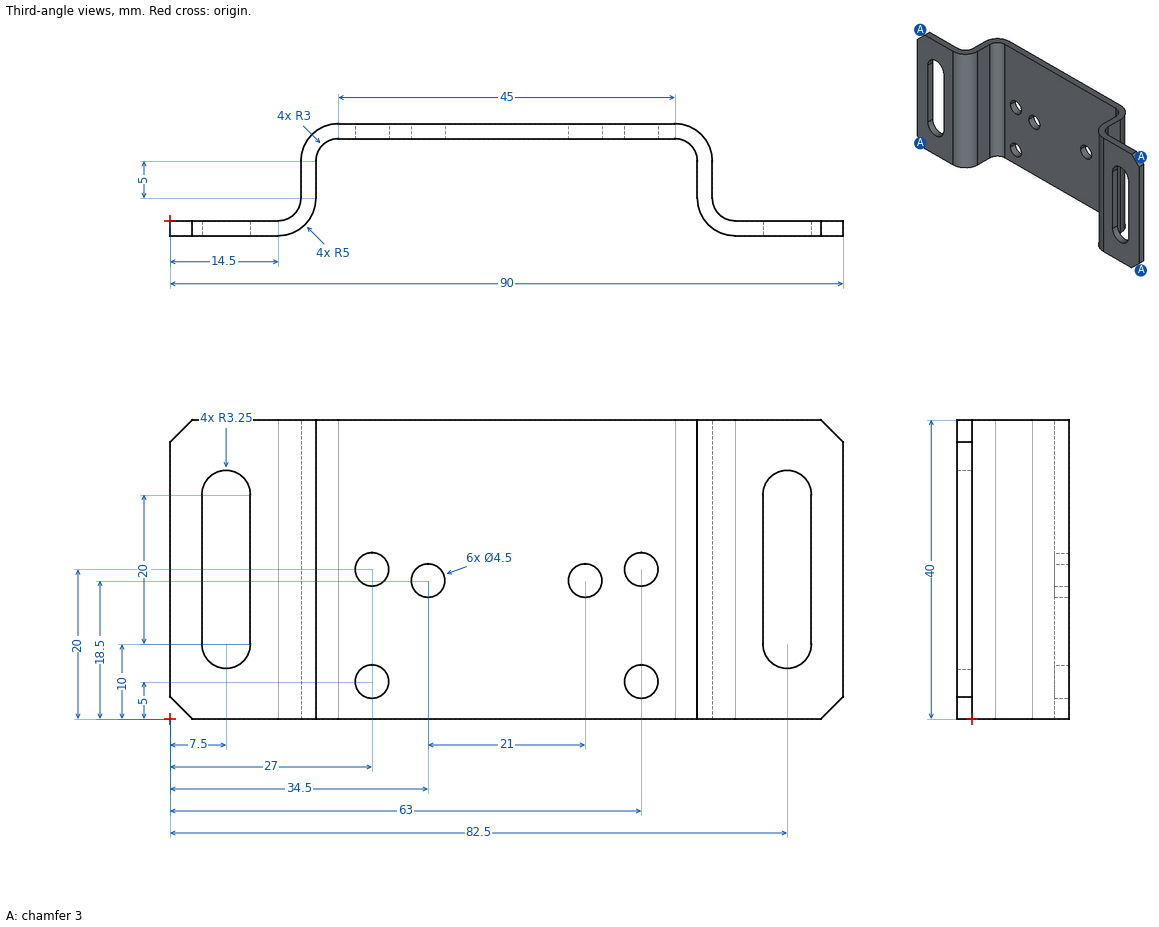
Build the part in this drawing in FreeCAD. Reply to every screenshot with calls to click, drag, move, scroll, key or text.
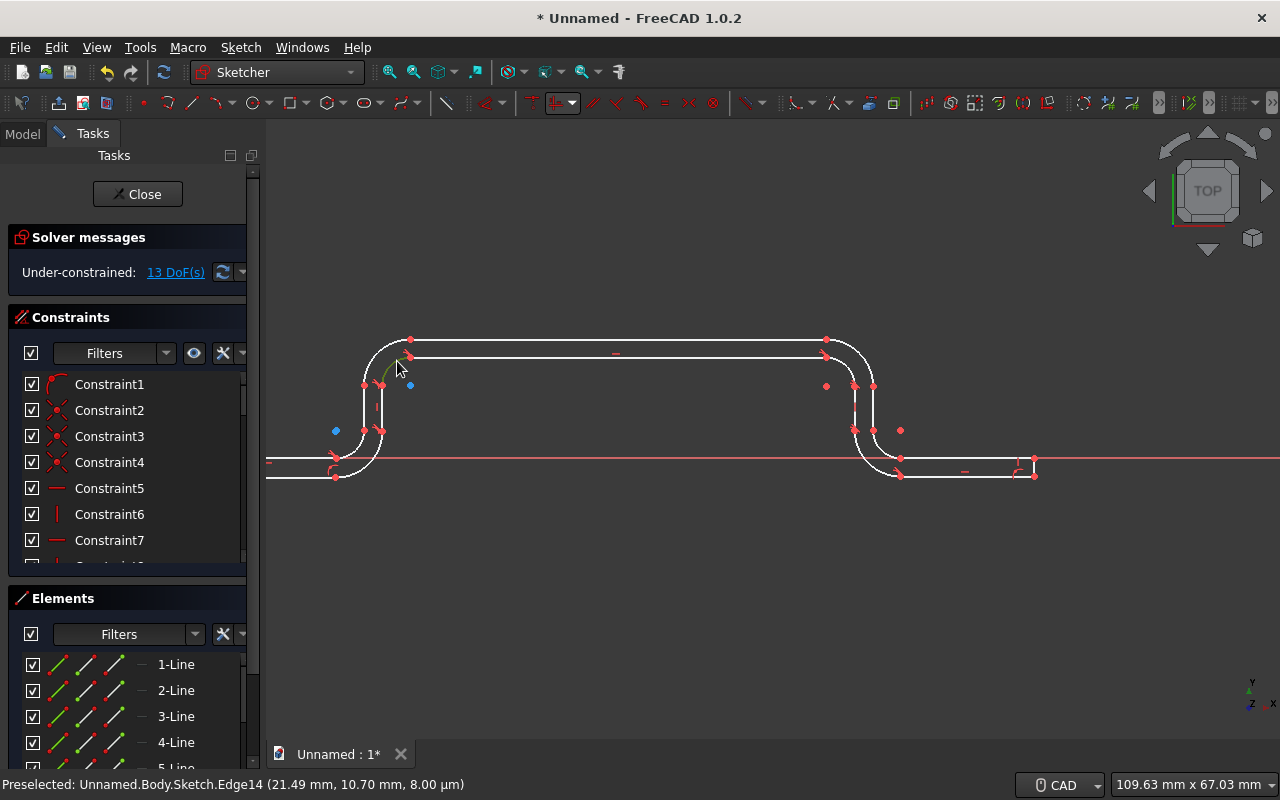
click(389, 345)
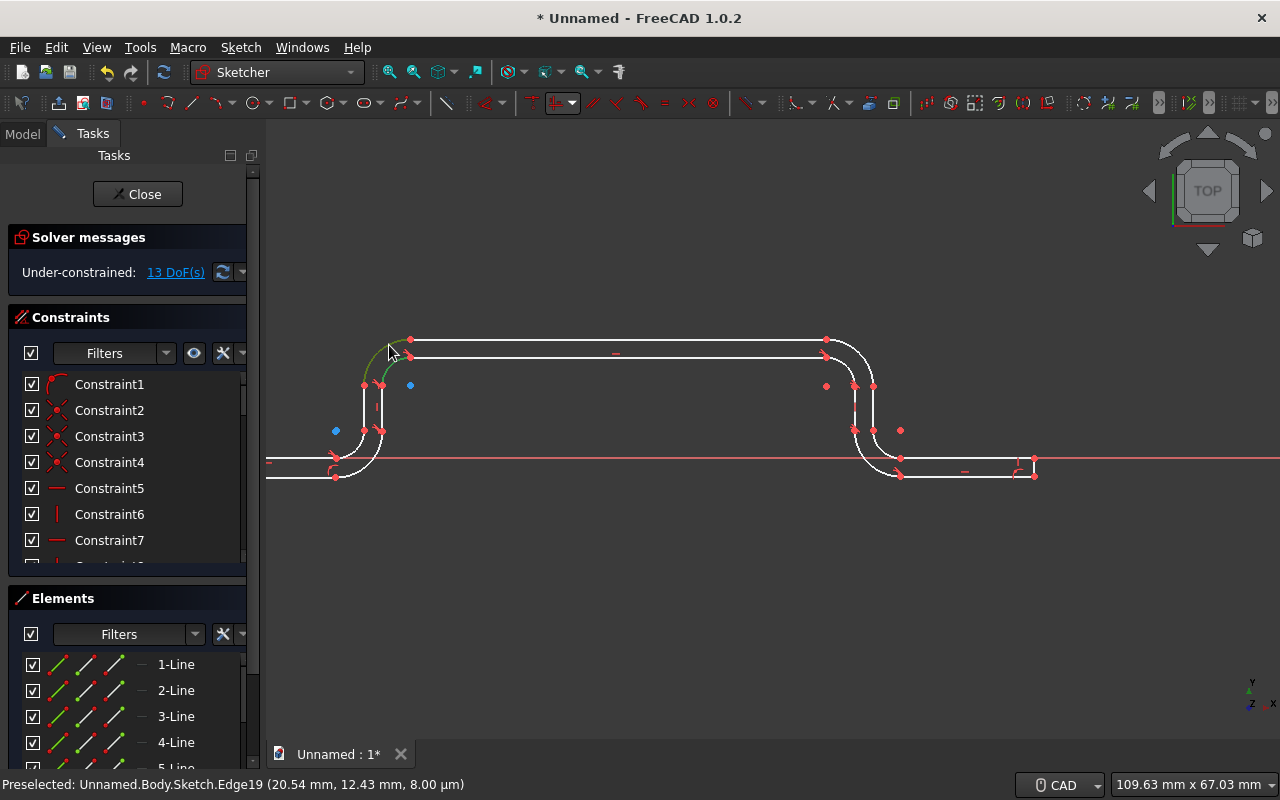
key(c)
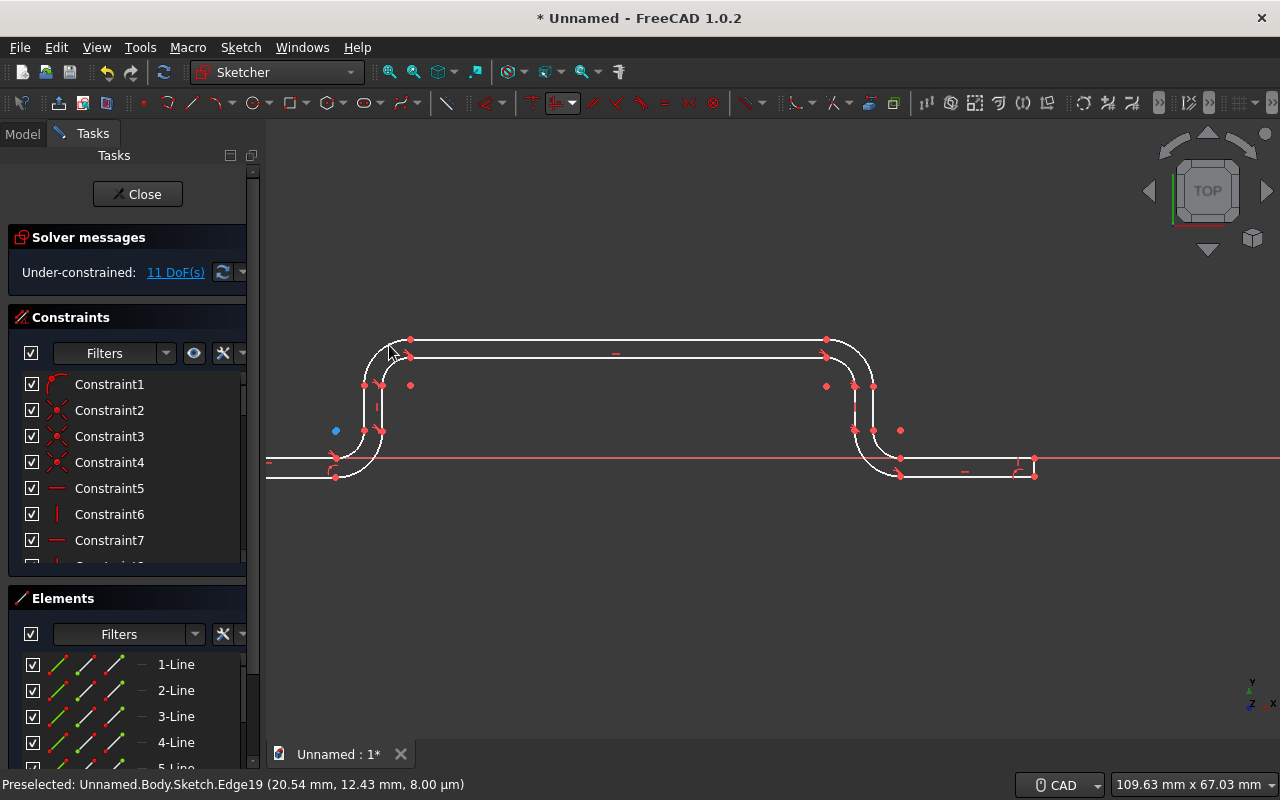
click(357, 473)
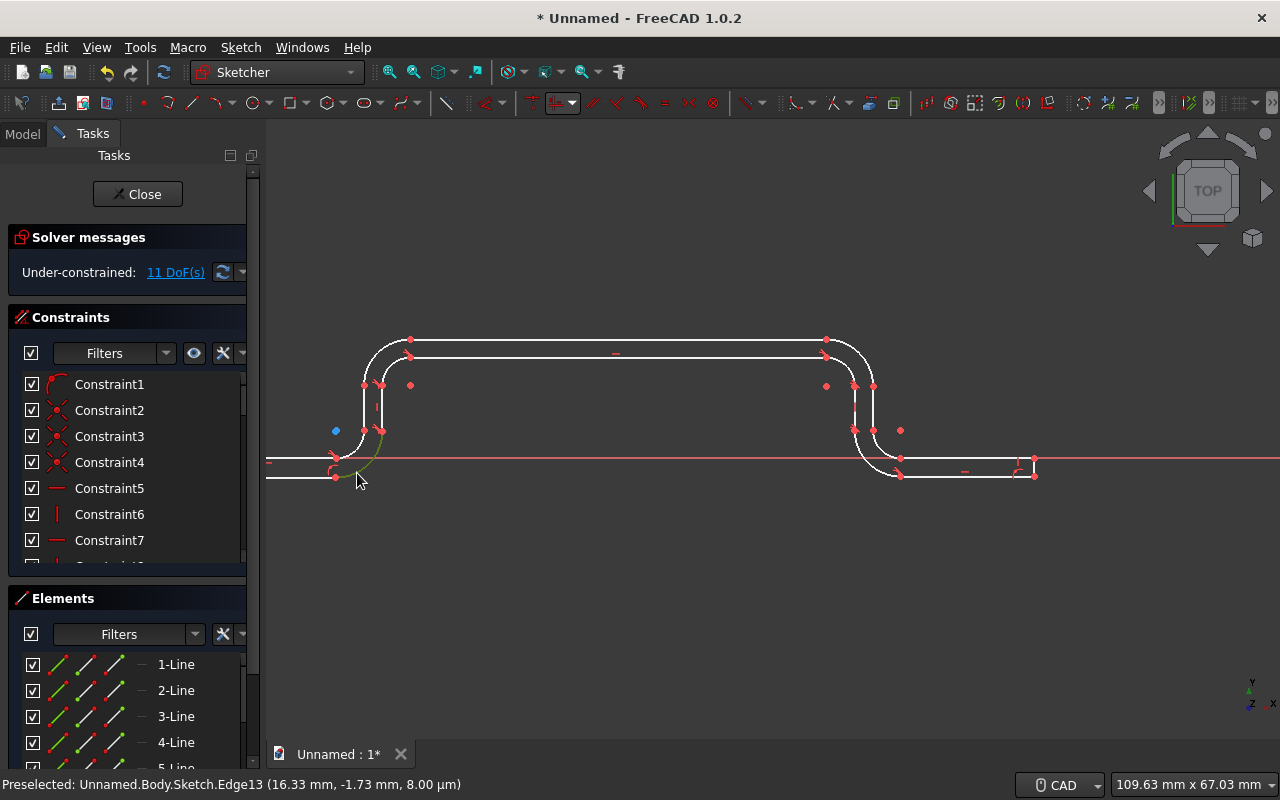
click(349, 455)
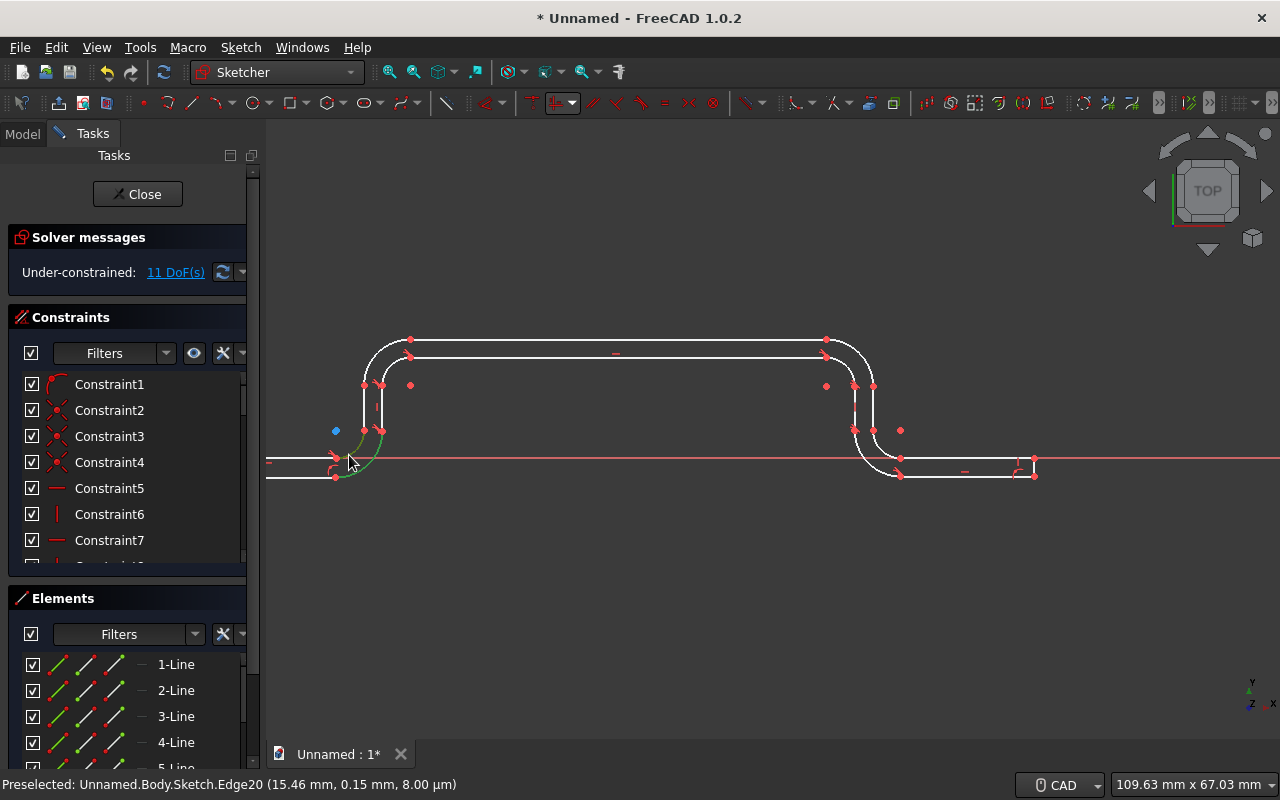
key(c)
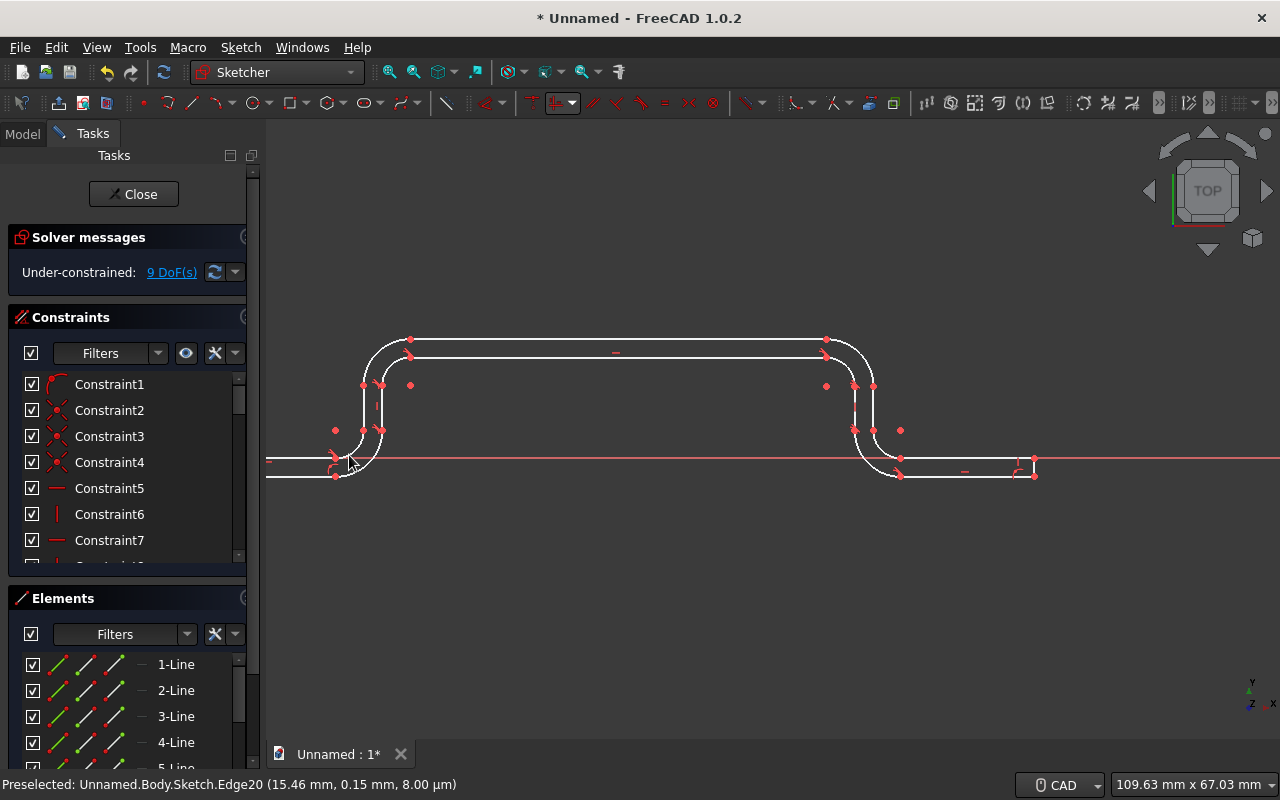
click(397, 361)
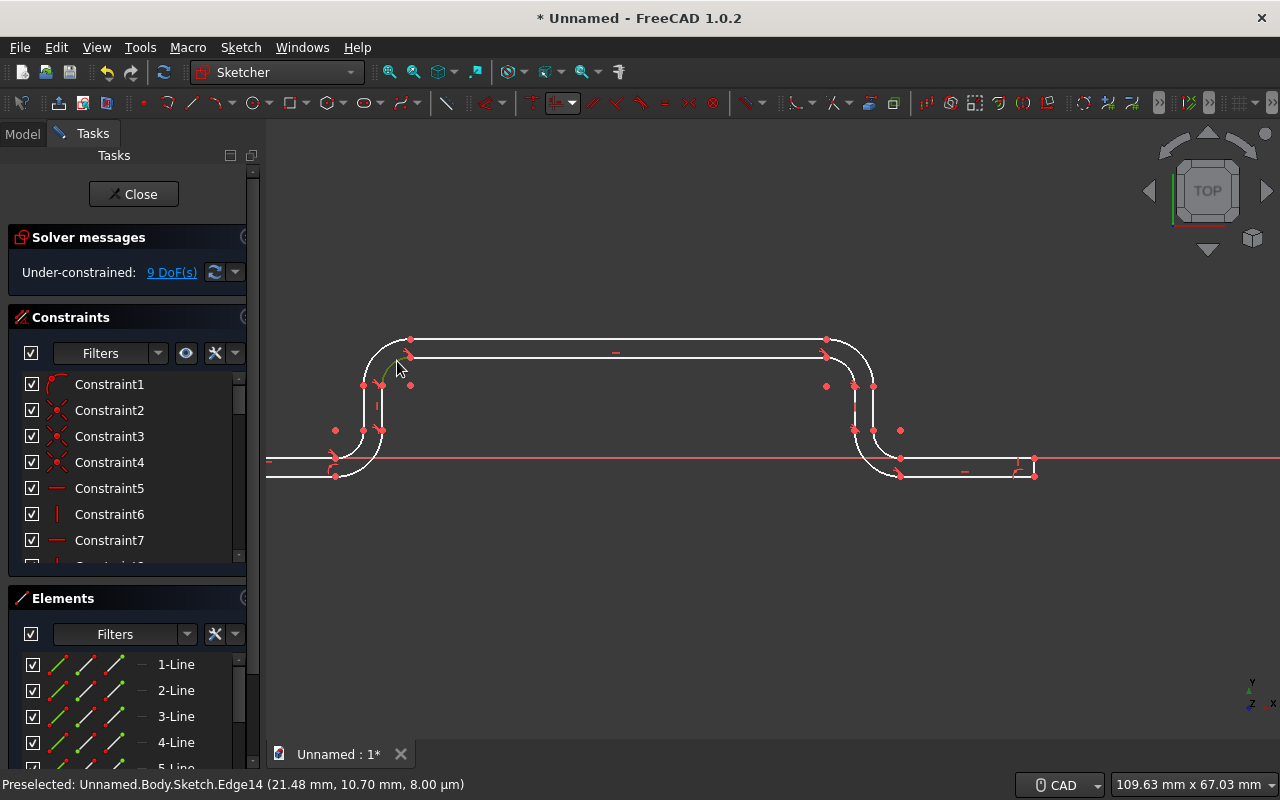
click(852, 373)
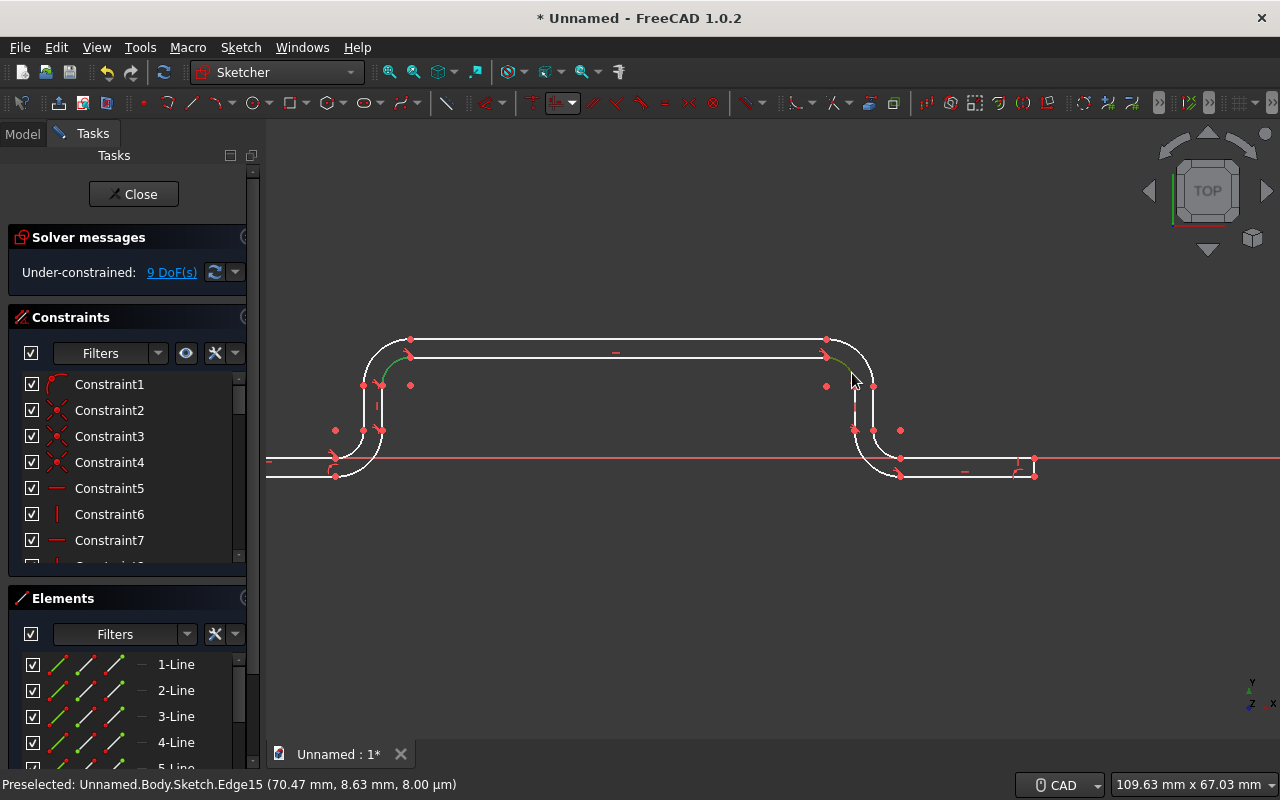
click(876, 443)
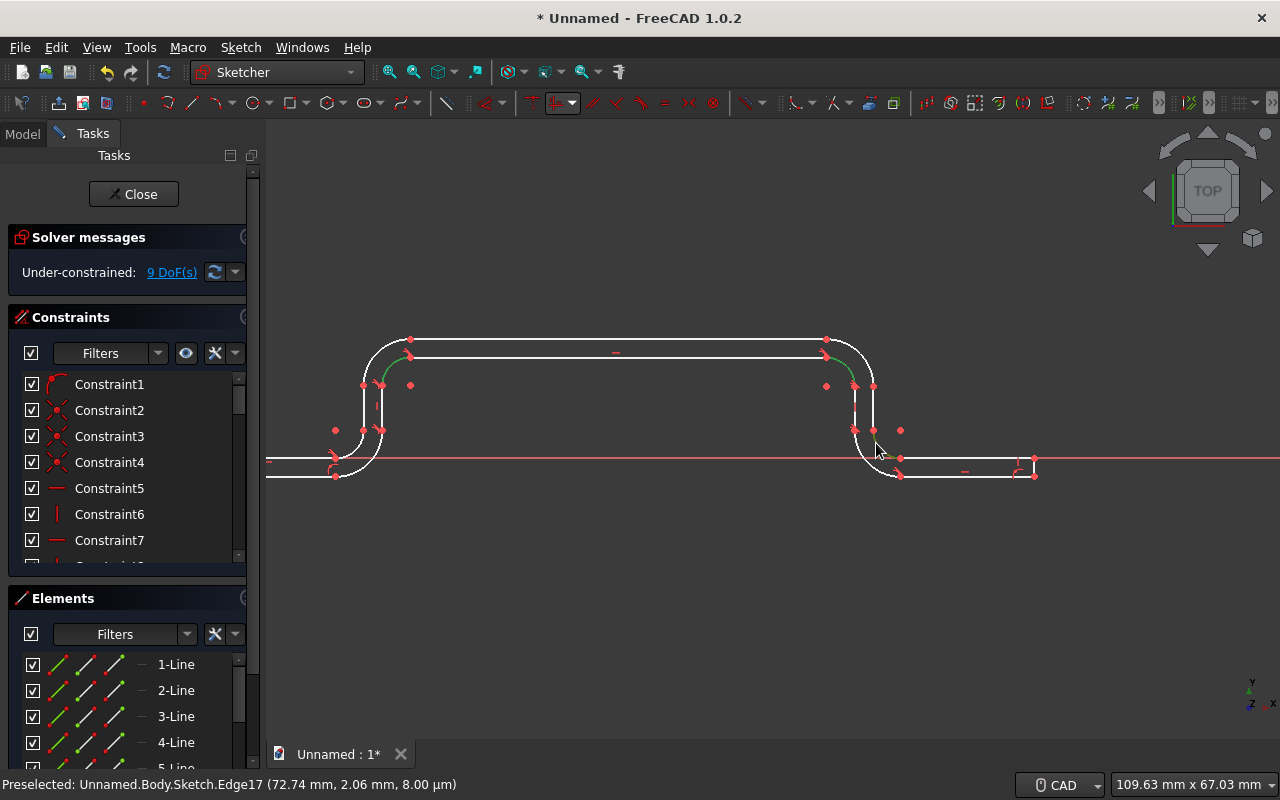
click(349, 455)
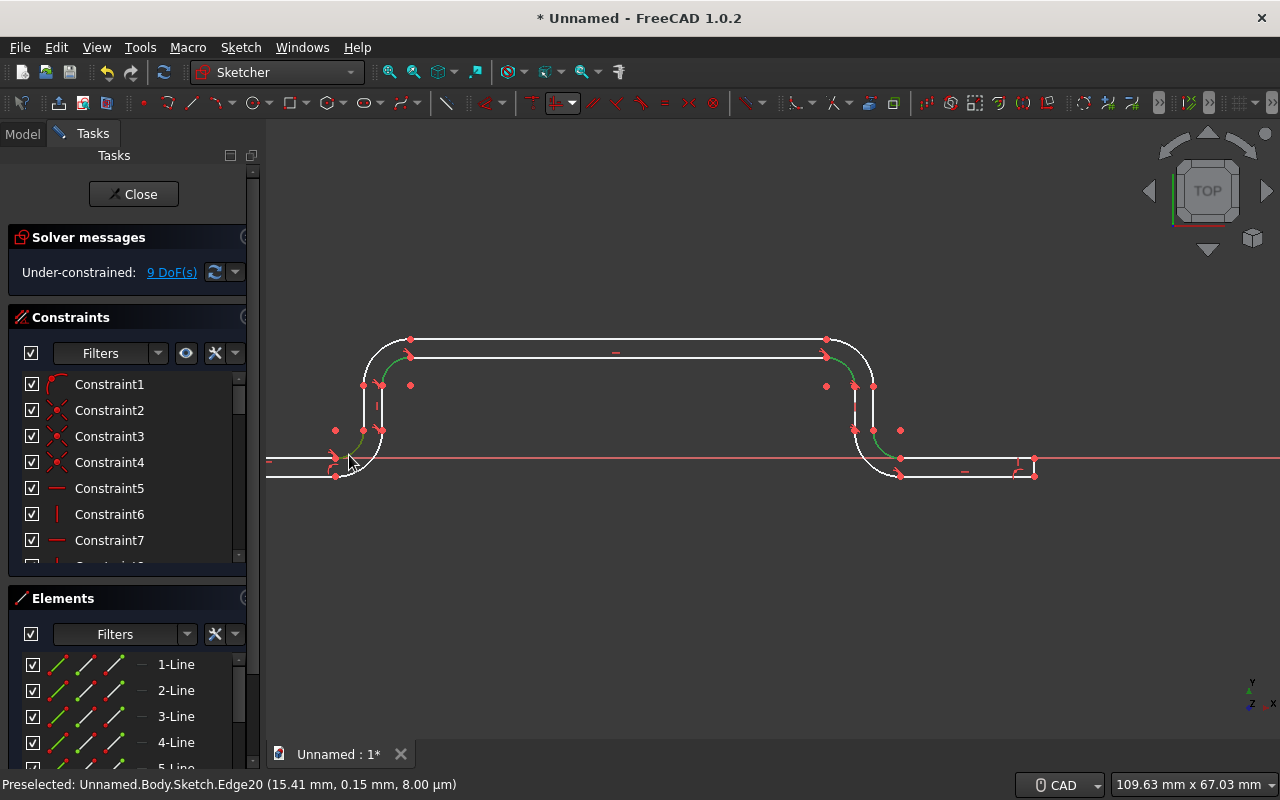
key(e)